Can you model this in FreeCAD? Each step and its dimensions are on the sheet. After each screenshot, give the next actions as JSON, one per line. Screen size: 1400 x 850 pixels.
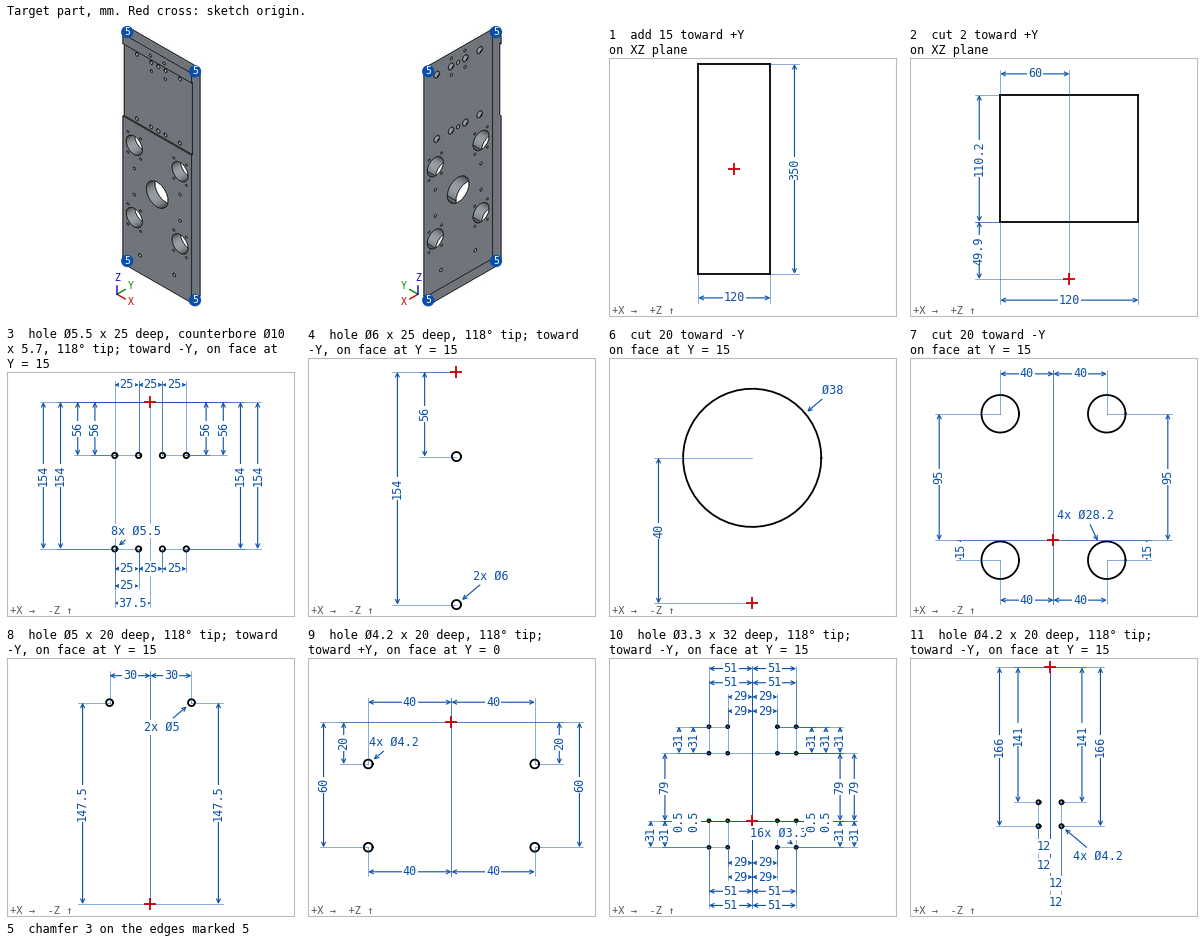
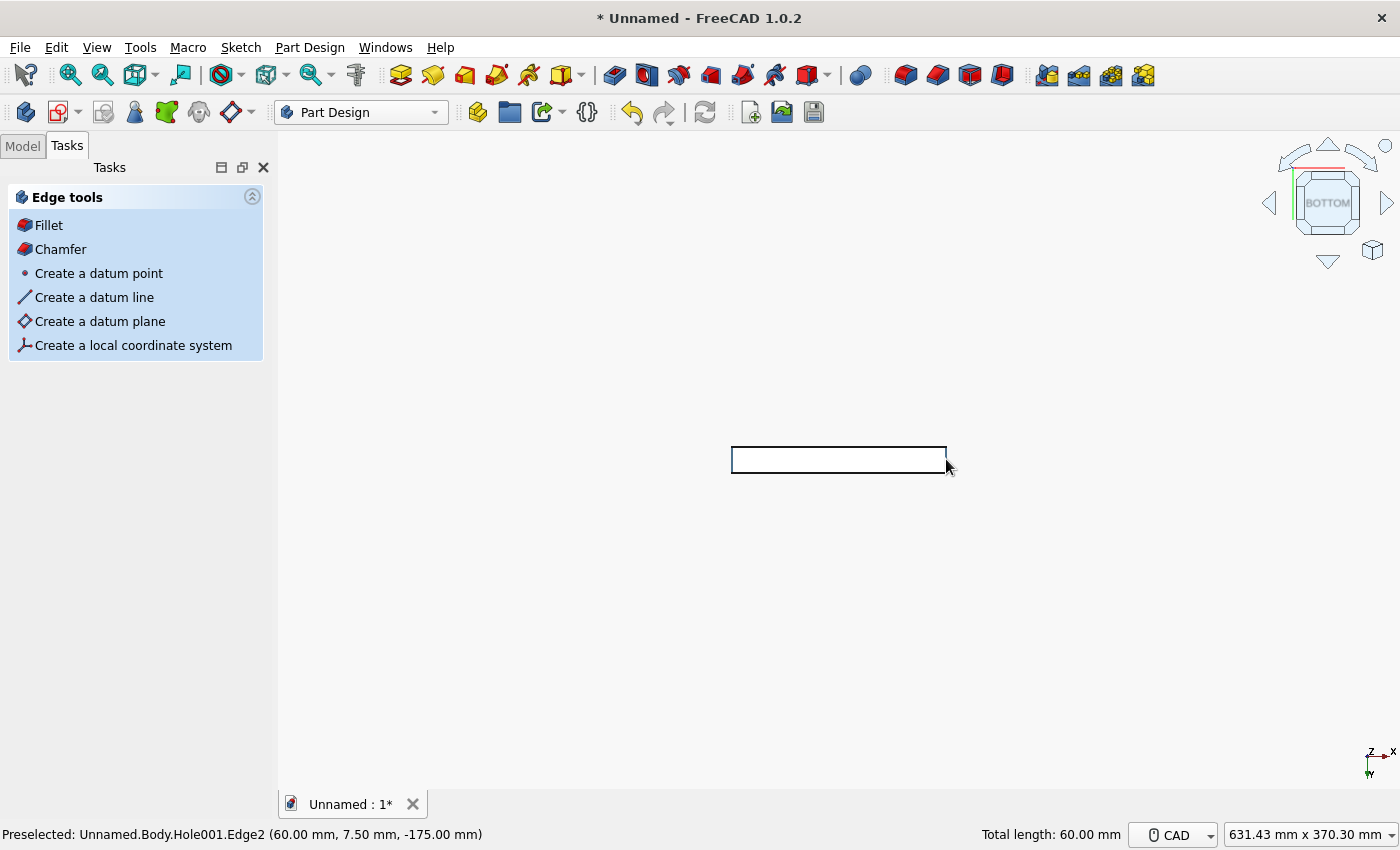
{"action": "left_click", "coordinate": [938, 76]}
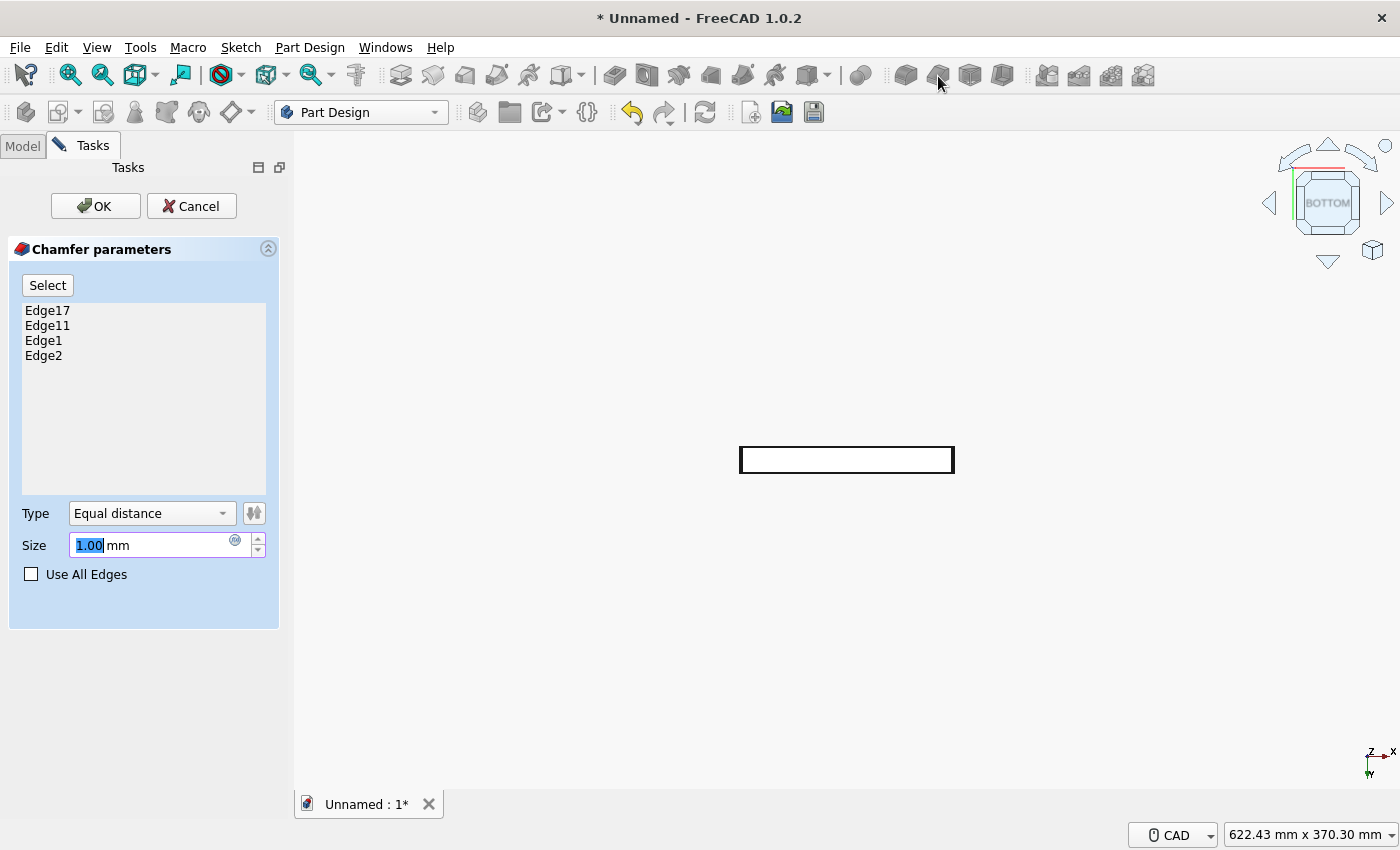
{"action": "type", "text": "3"}
{"action": "key", "text": "Tab"}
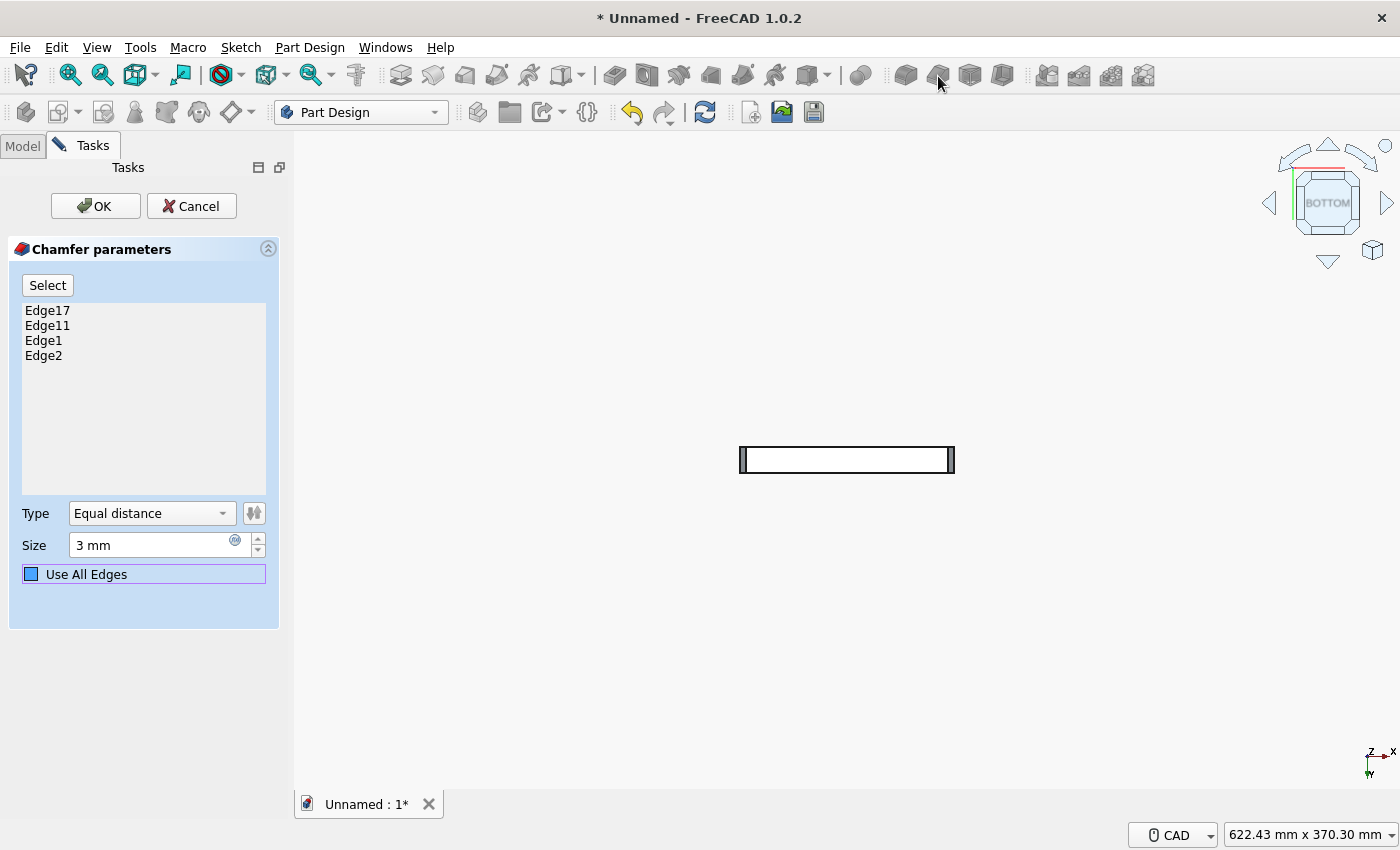
{"action": "left_click", "coordinate": [96, 206]}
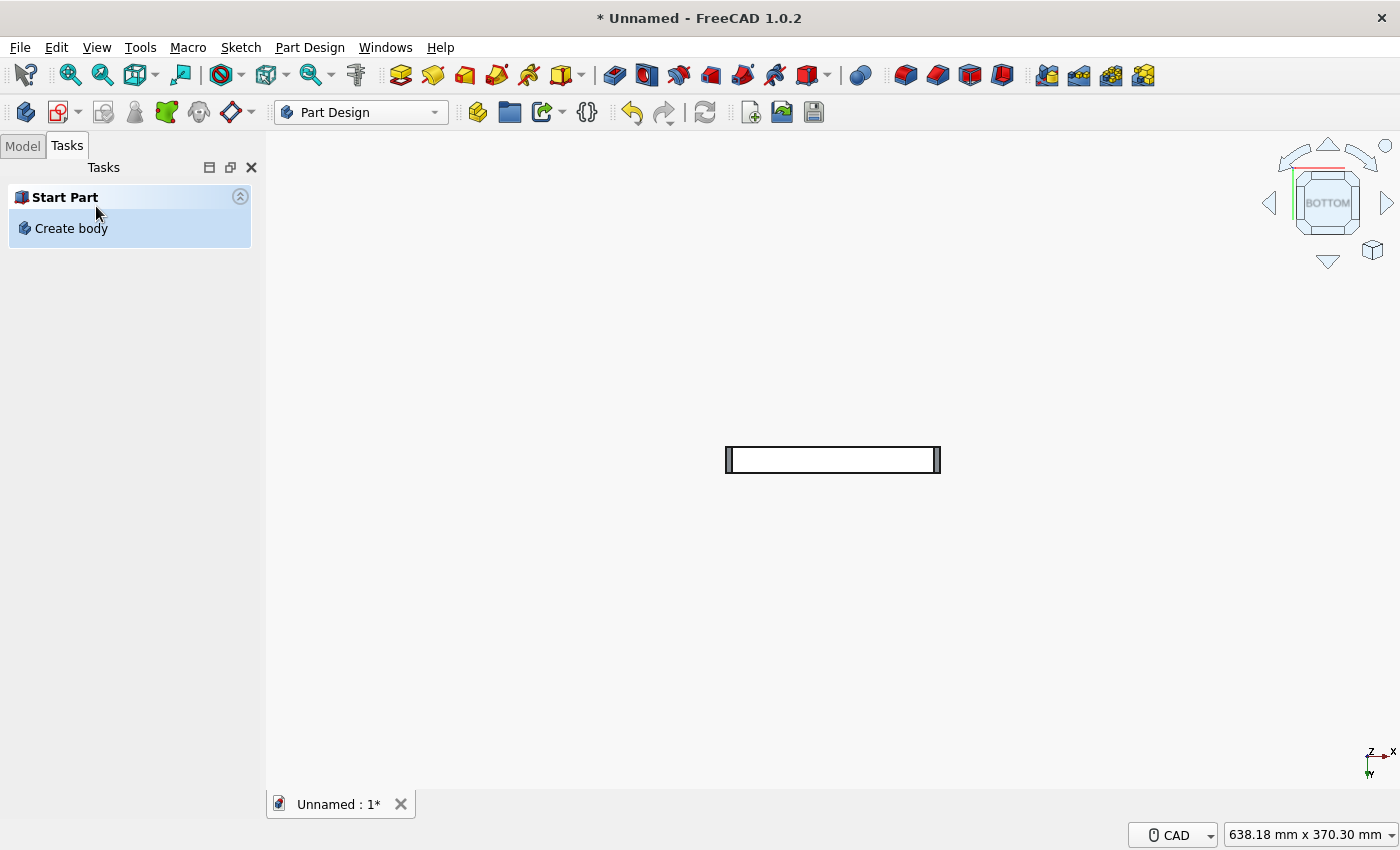
{"action": "left_click", "coordinate": [72, 76]}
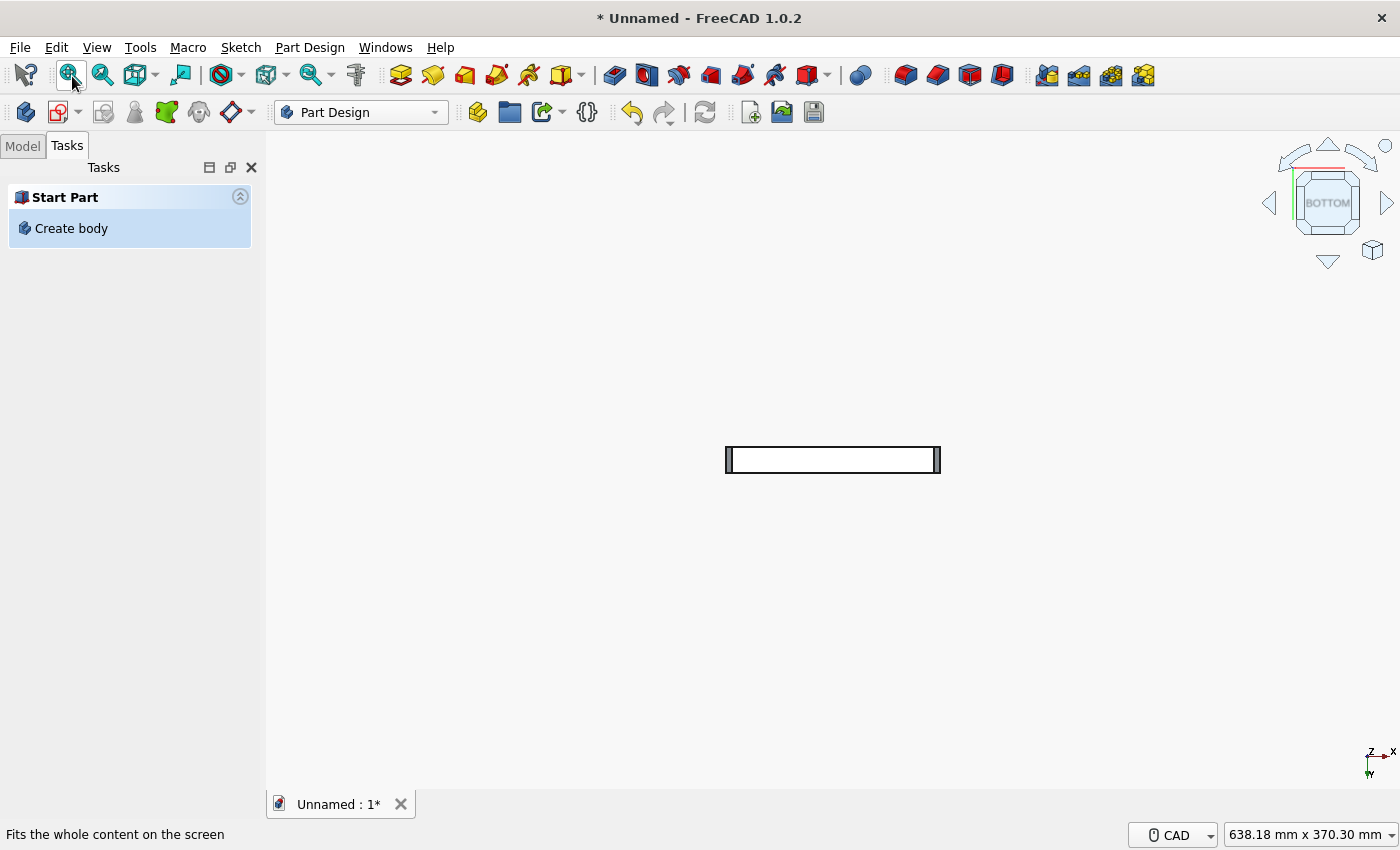
{"action": "key", "text": "4"}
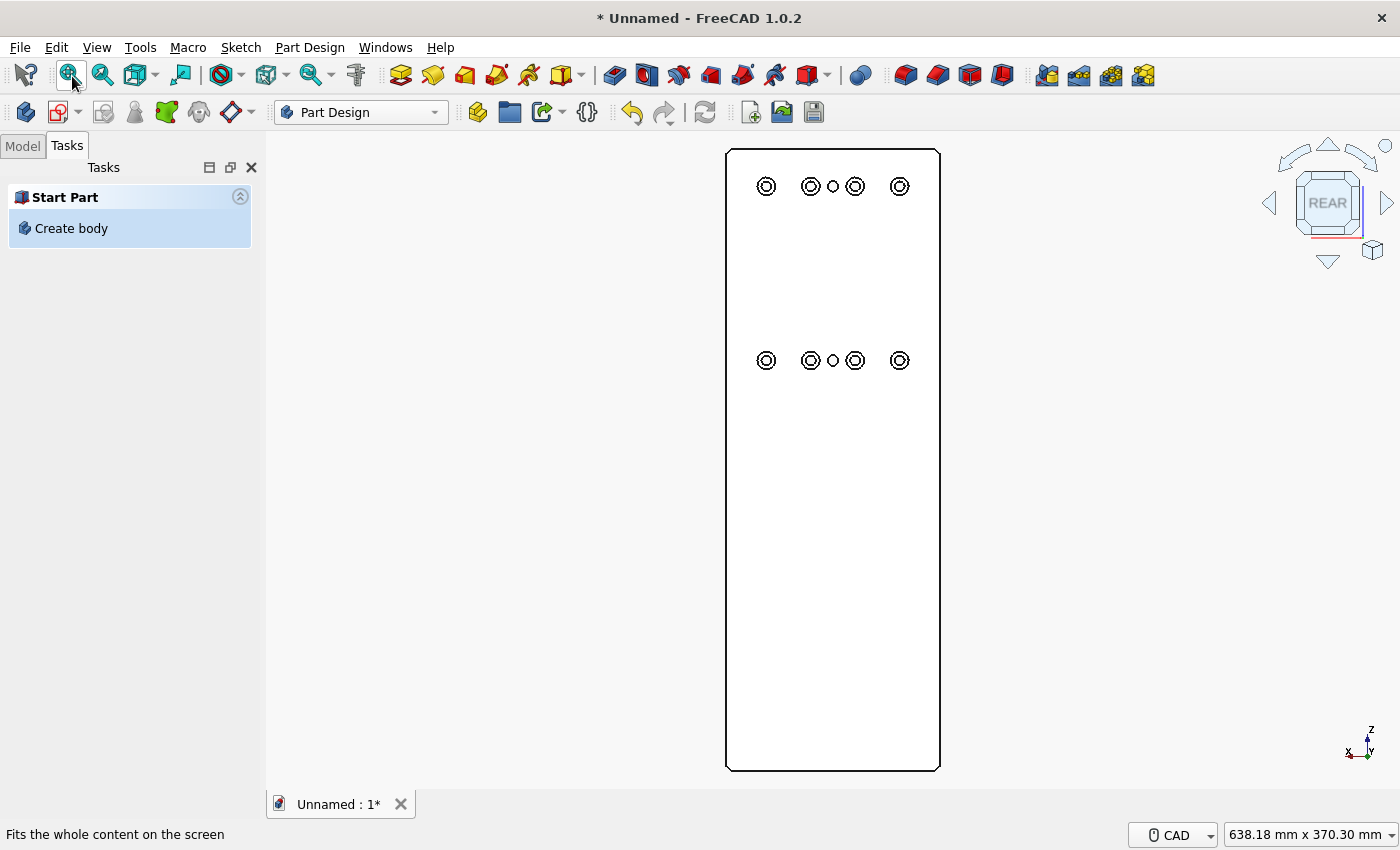
{"action": "left_click", "coordinate": [833, 548]}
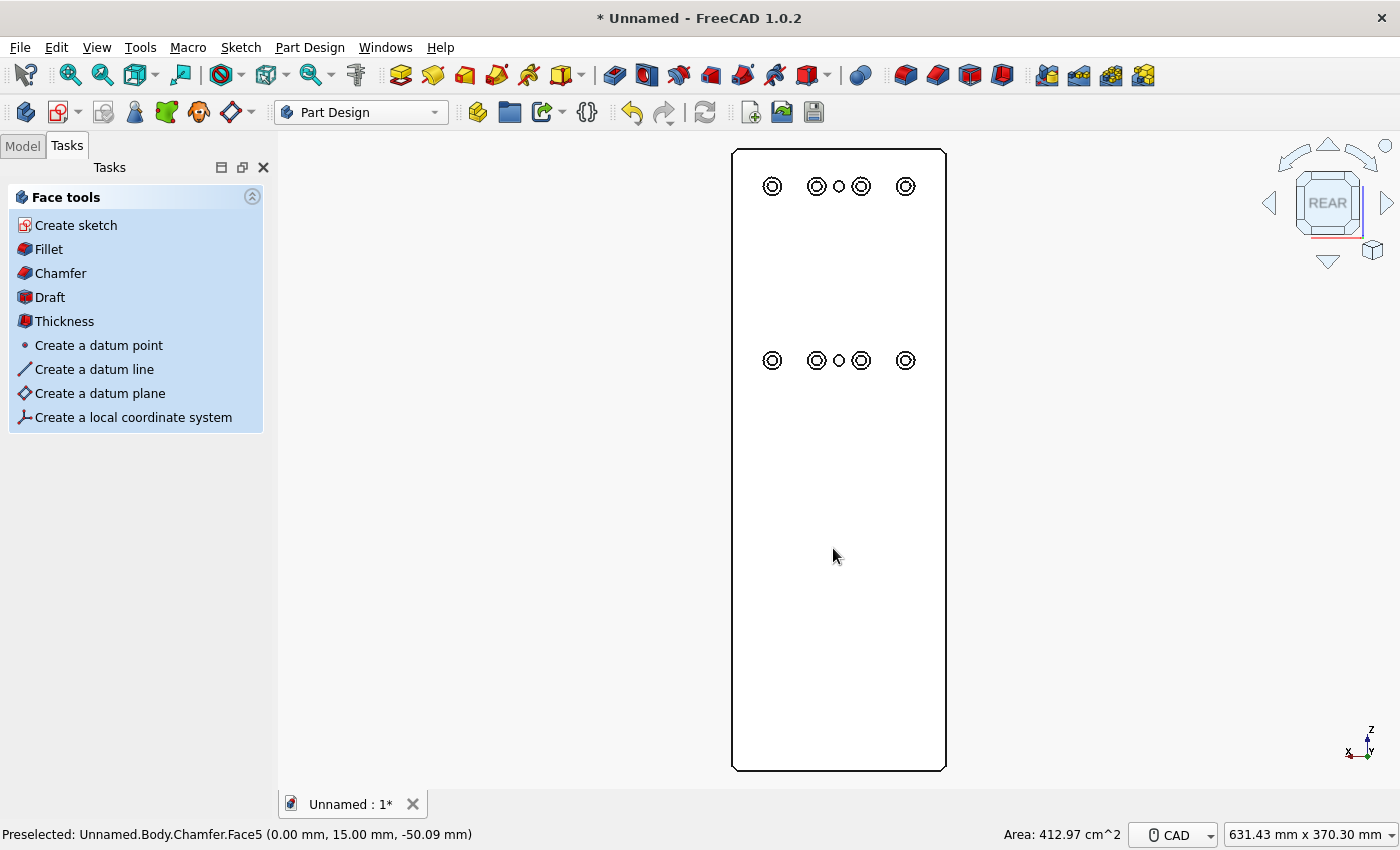
{"action": "left_click", "coordinate": [58, 112]}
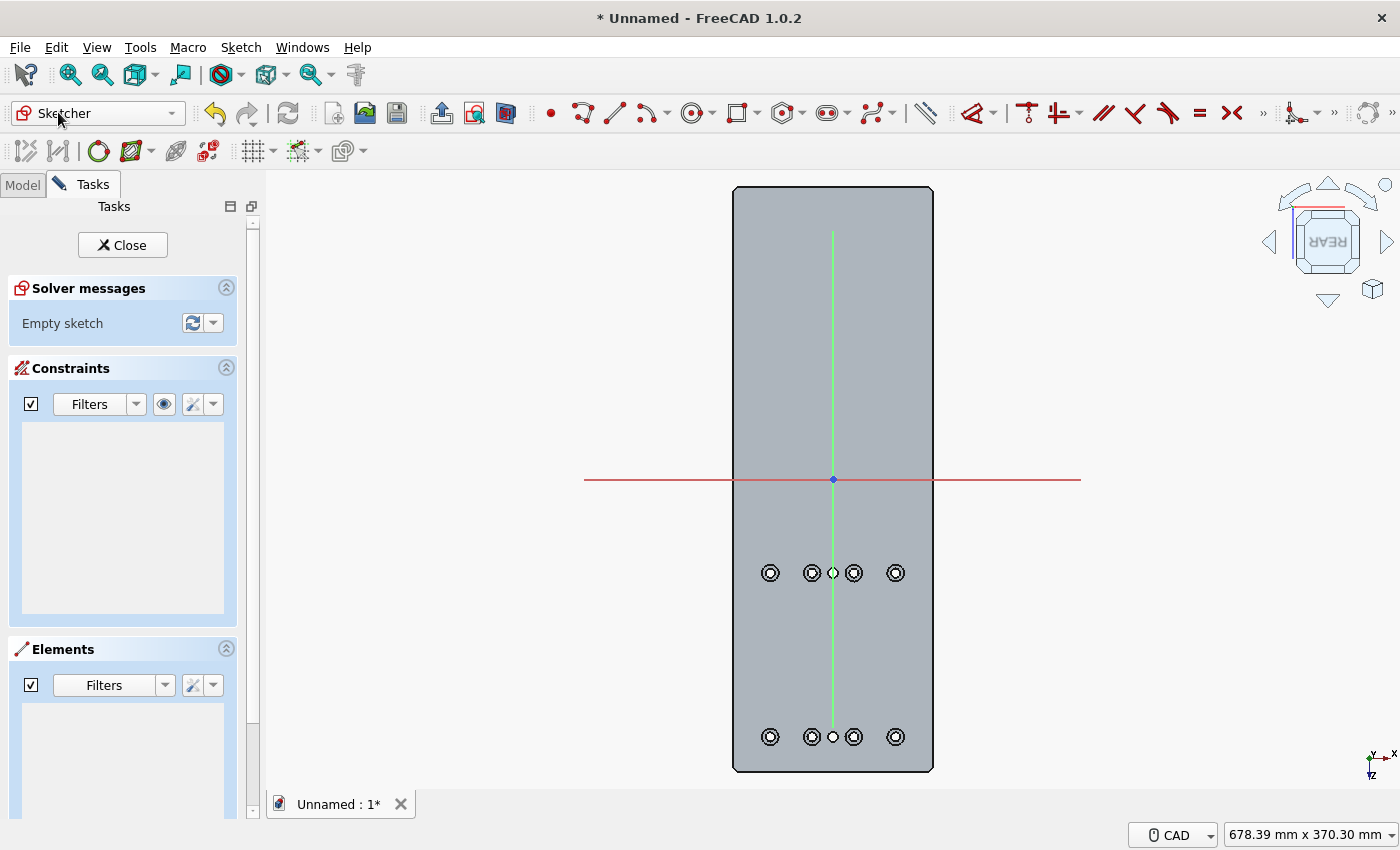
{"action": "scroll", "coordinate": [855, 414], "scroll_direction": "up", "scroll_amount": 7}